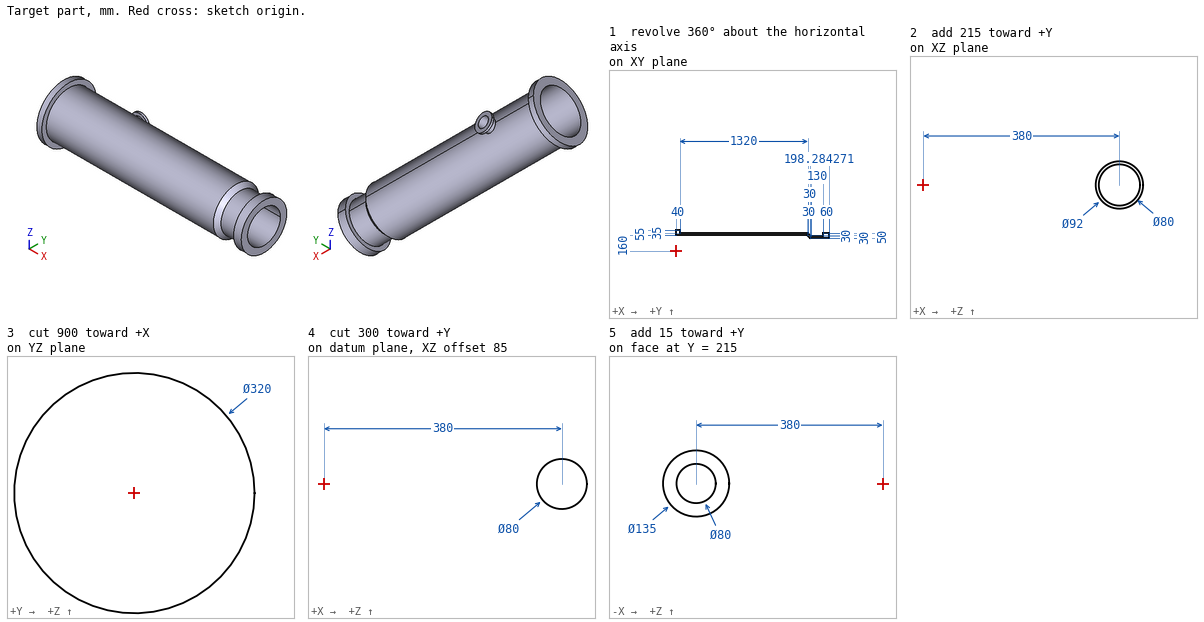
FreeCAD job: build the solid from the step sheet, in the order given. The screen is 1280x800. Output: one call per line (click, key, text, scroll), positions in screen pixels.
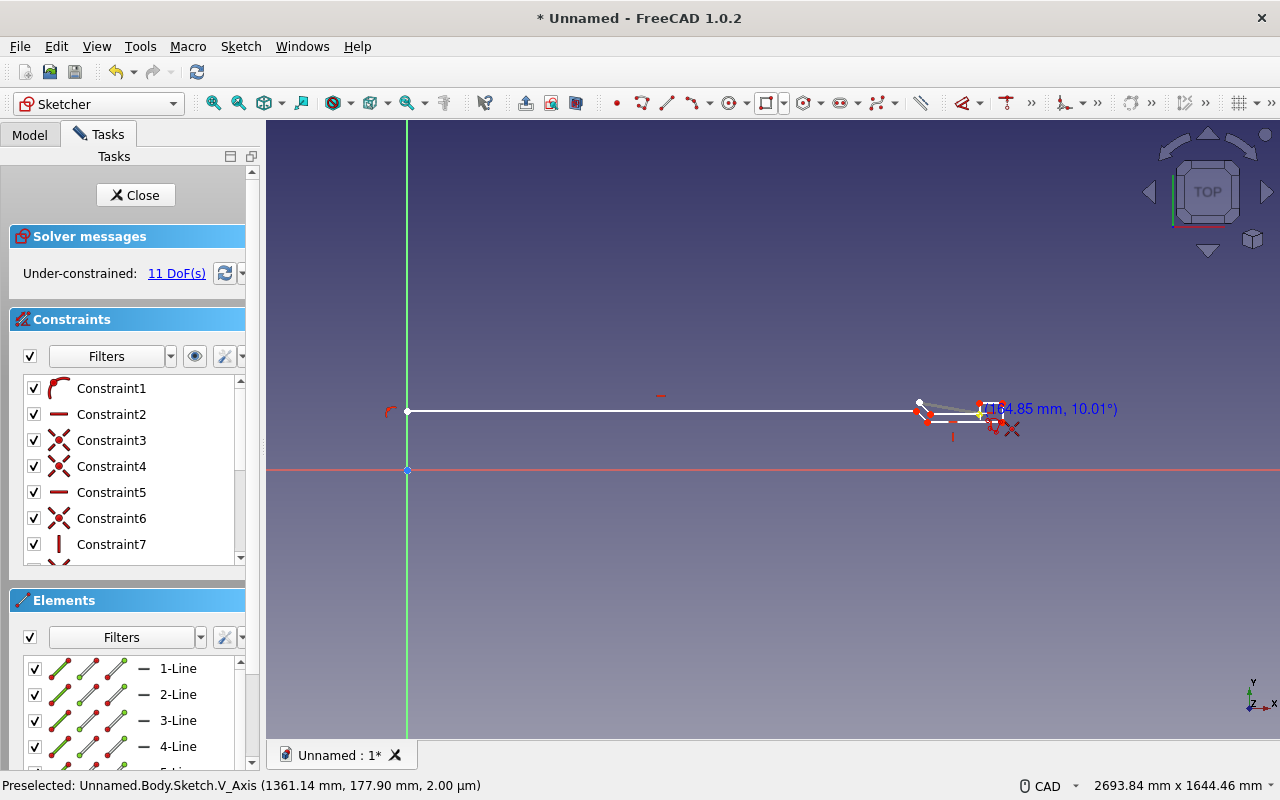
scroll(422, 403, up, 4)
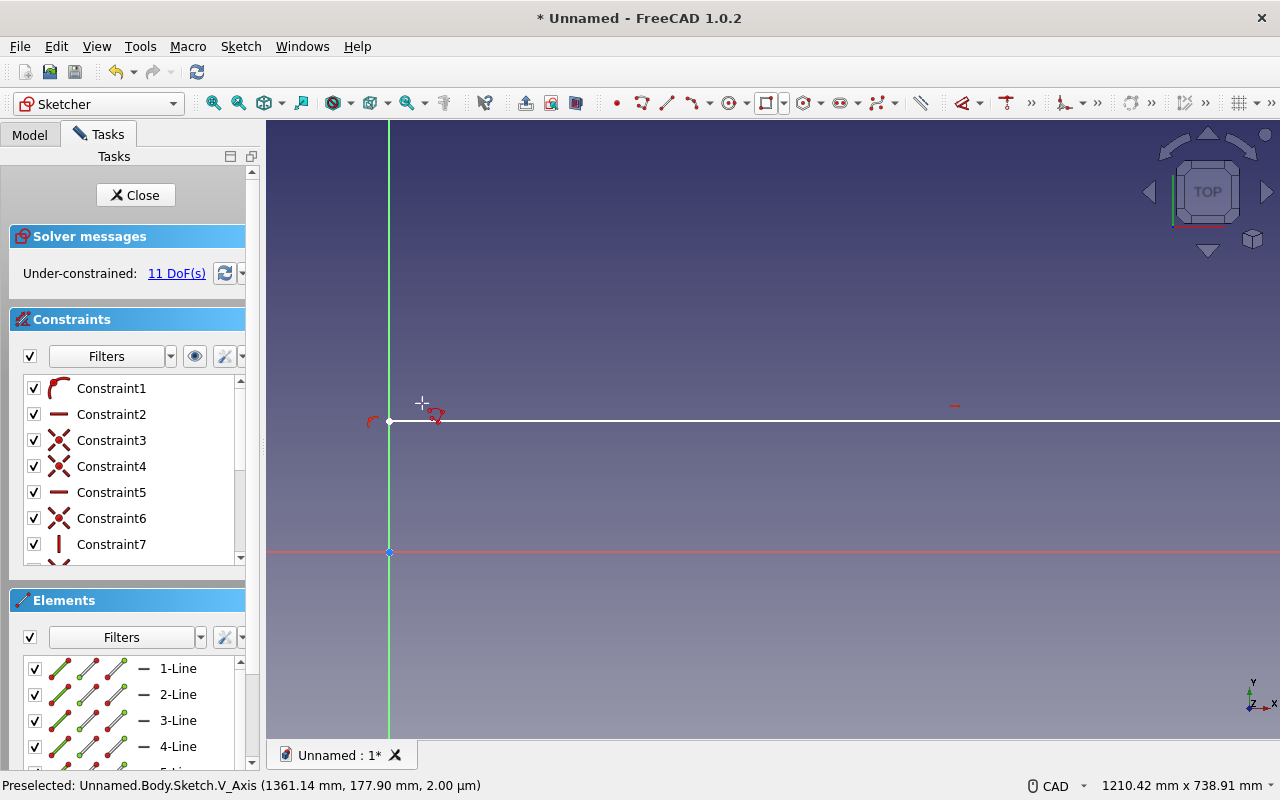
click(423, 401)
click(423, 372)
click(398, 372)
click(389, 421)
key(Escape)
key(Escape)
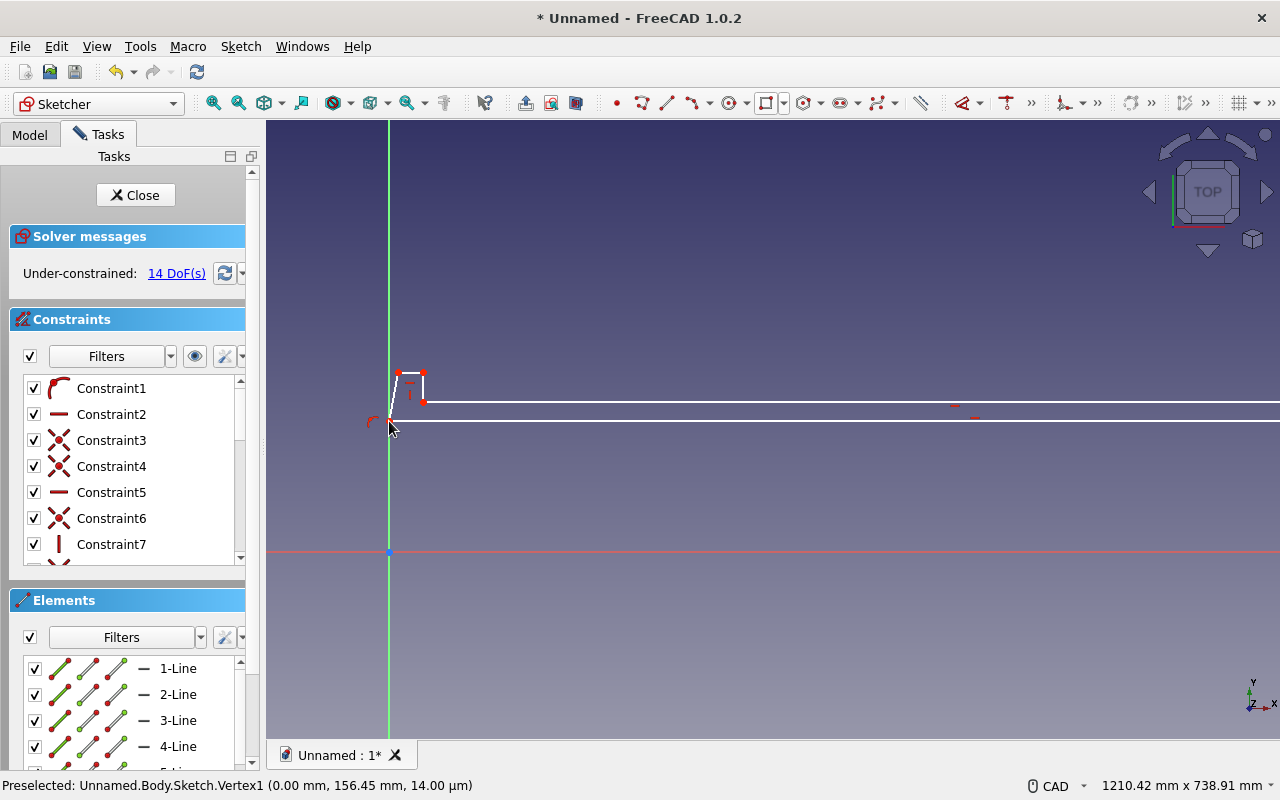
click(392, 407)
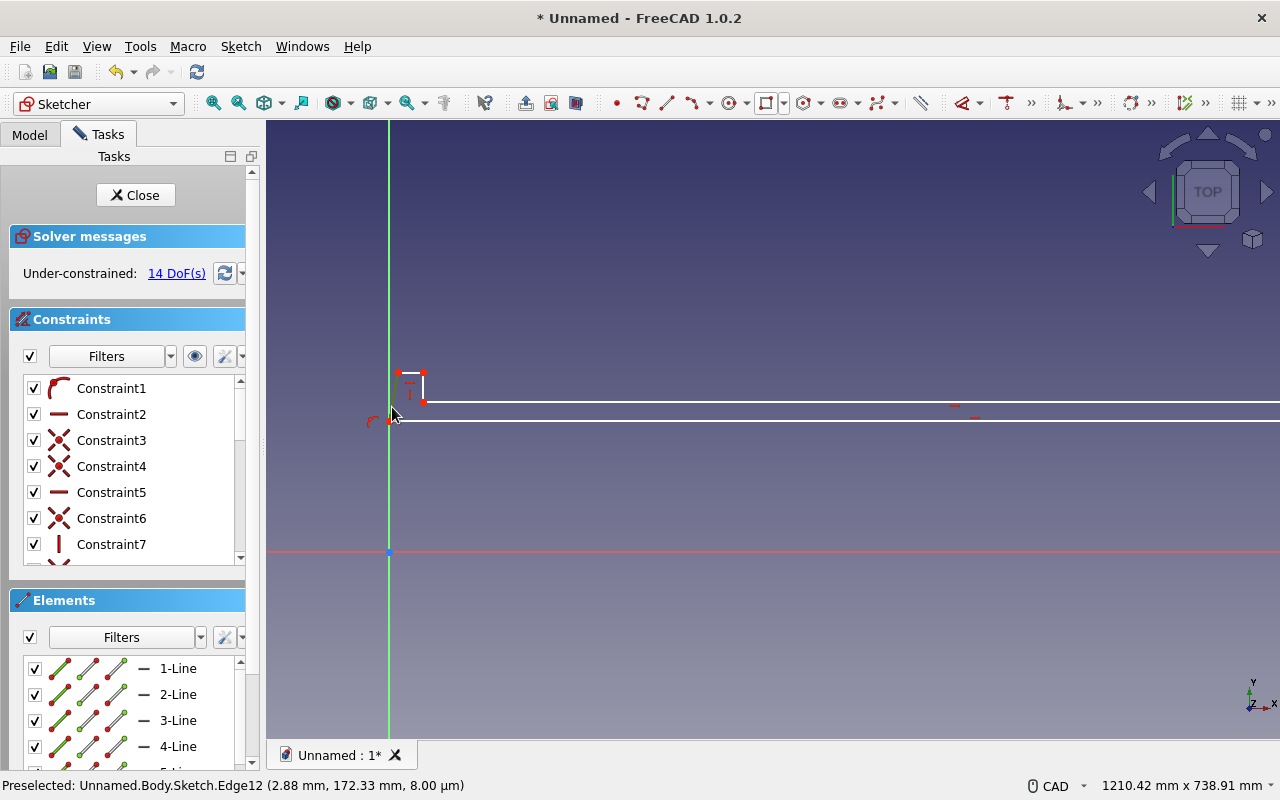
key(v)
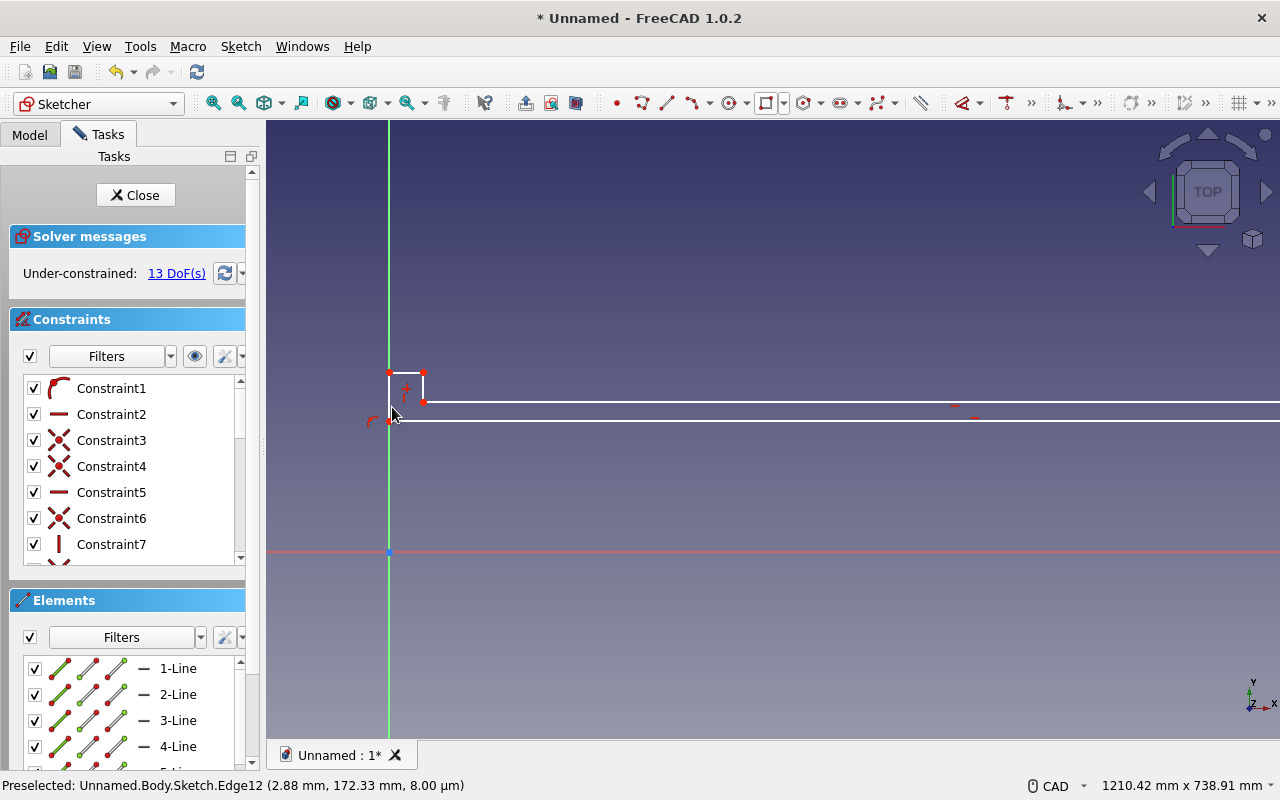
scroll(422, 403, down, 4)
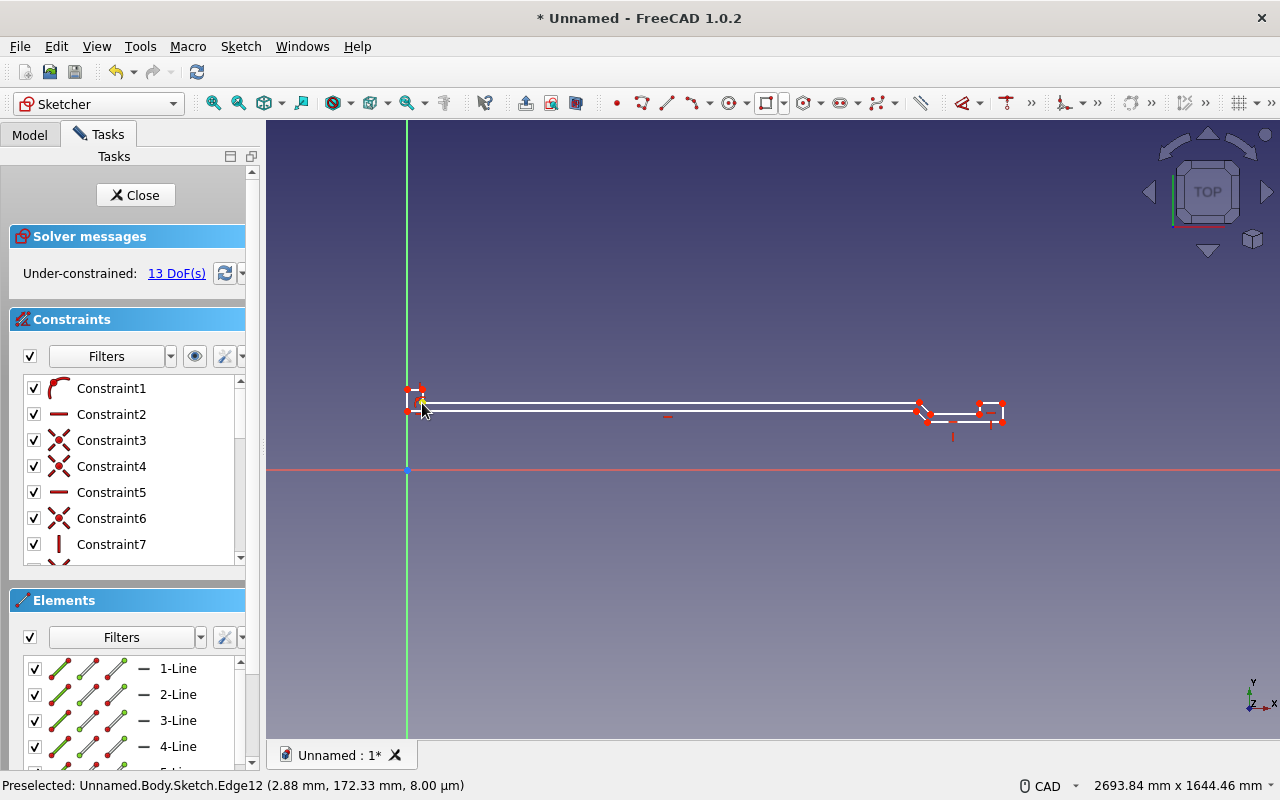
scroll(1003, 417, up, 5)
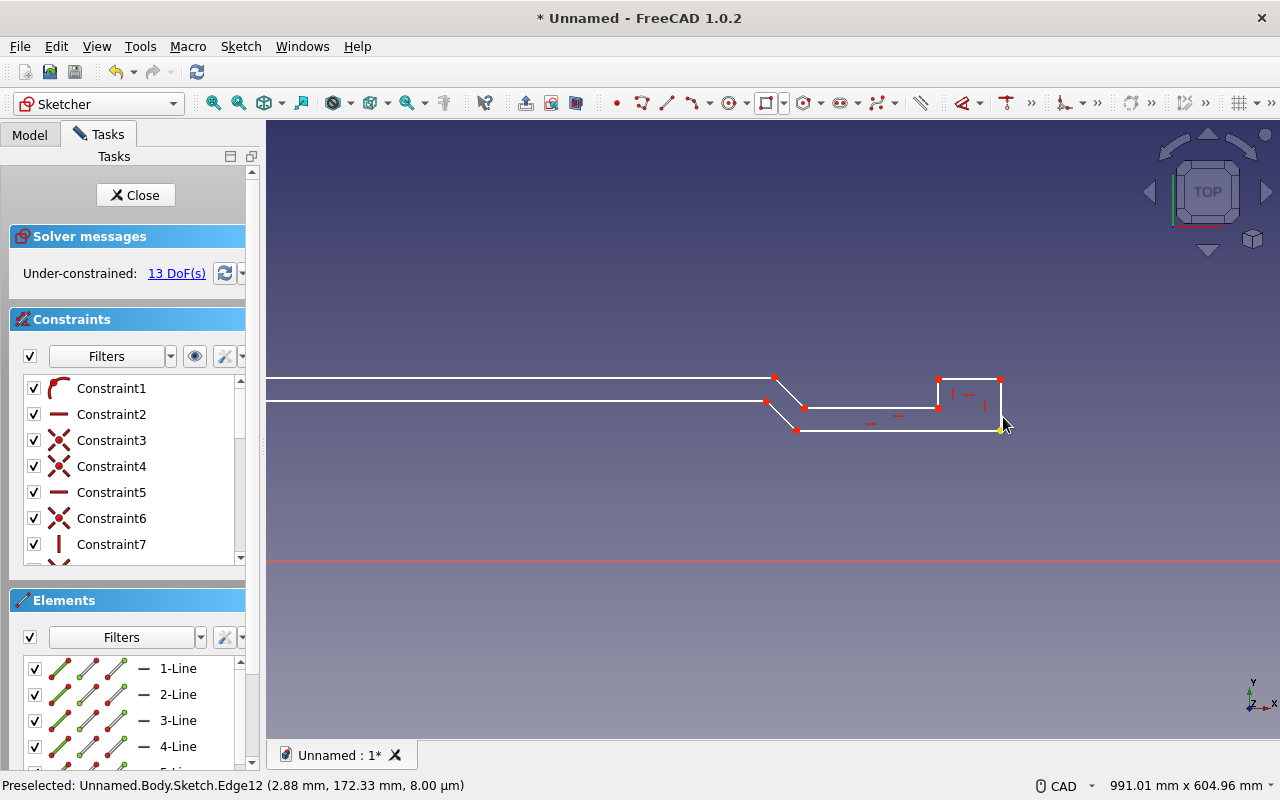
click(1001, 415)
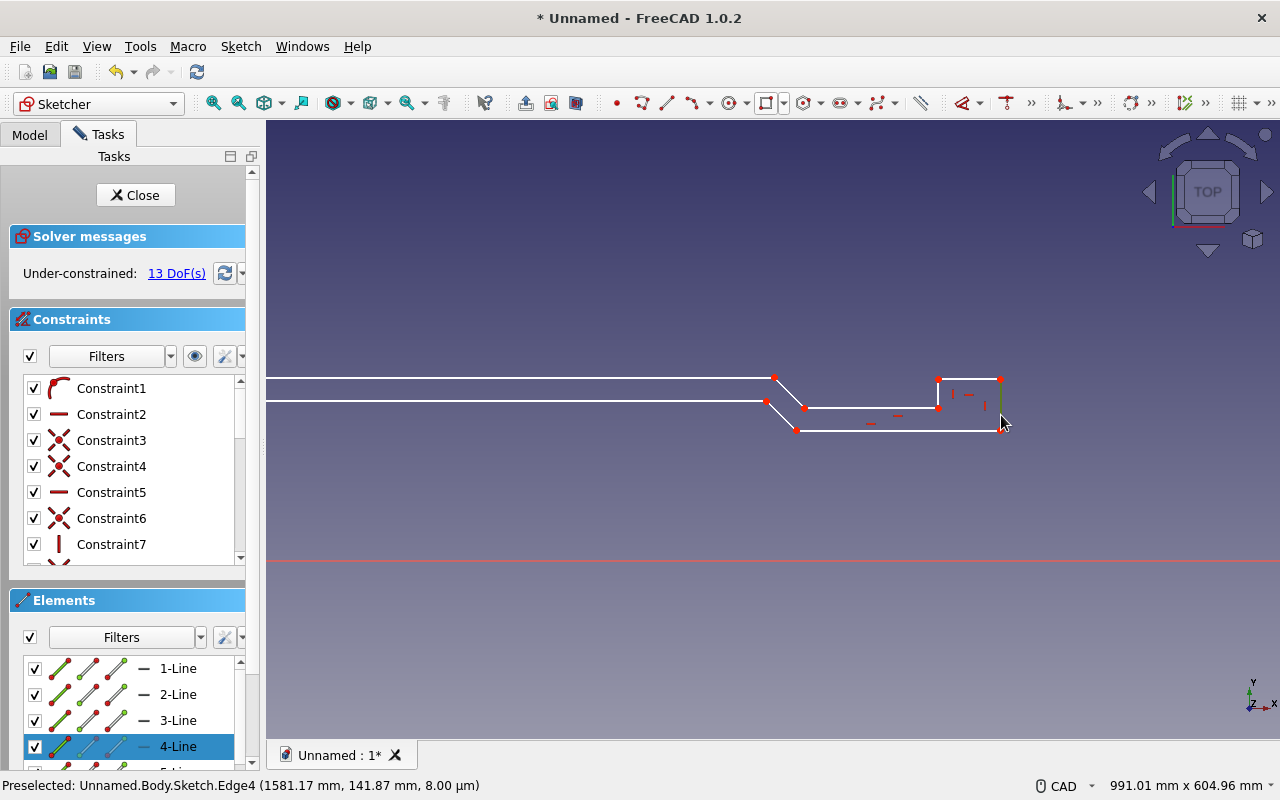
key(i)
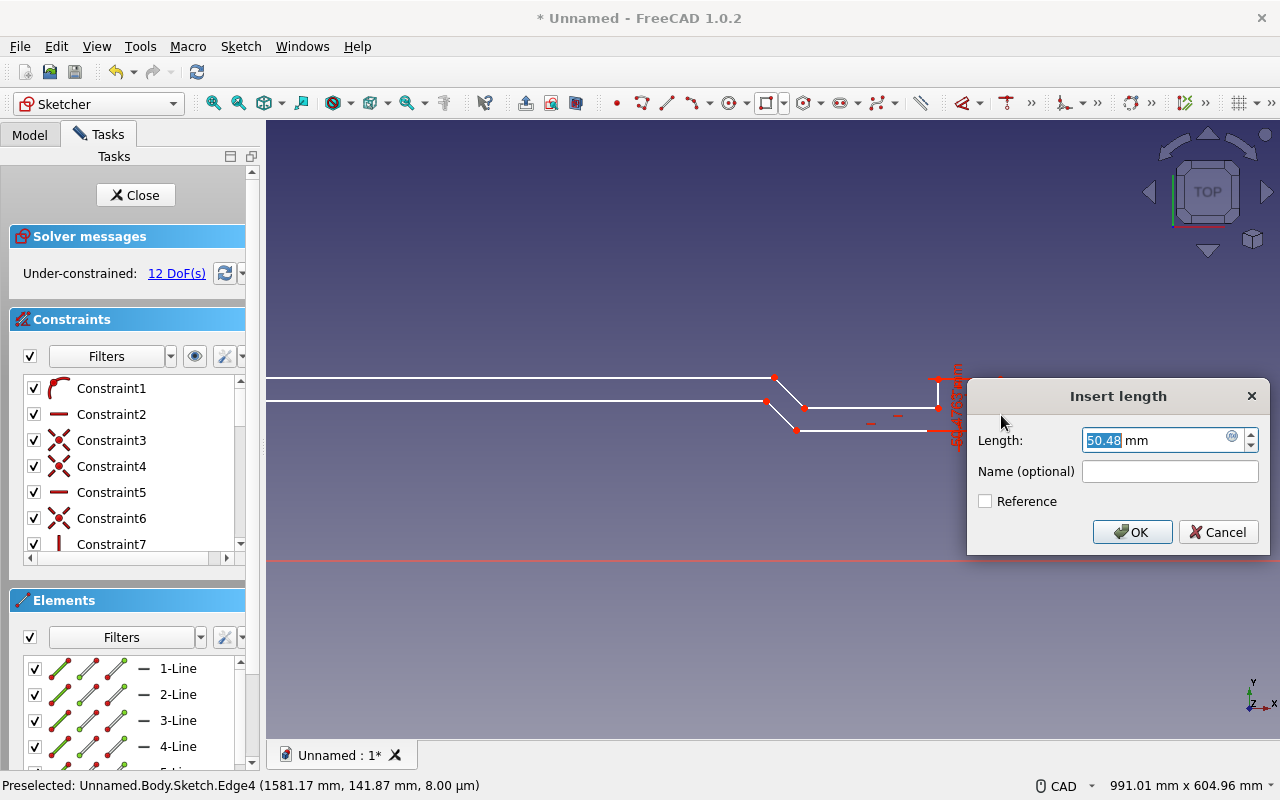
text(50)
key(Return)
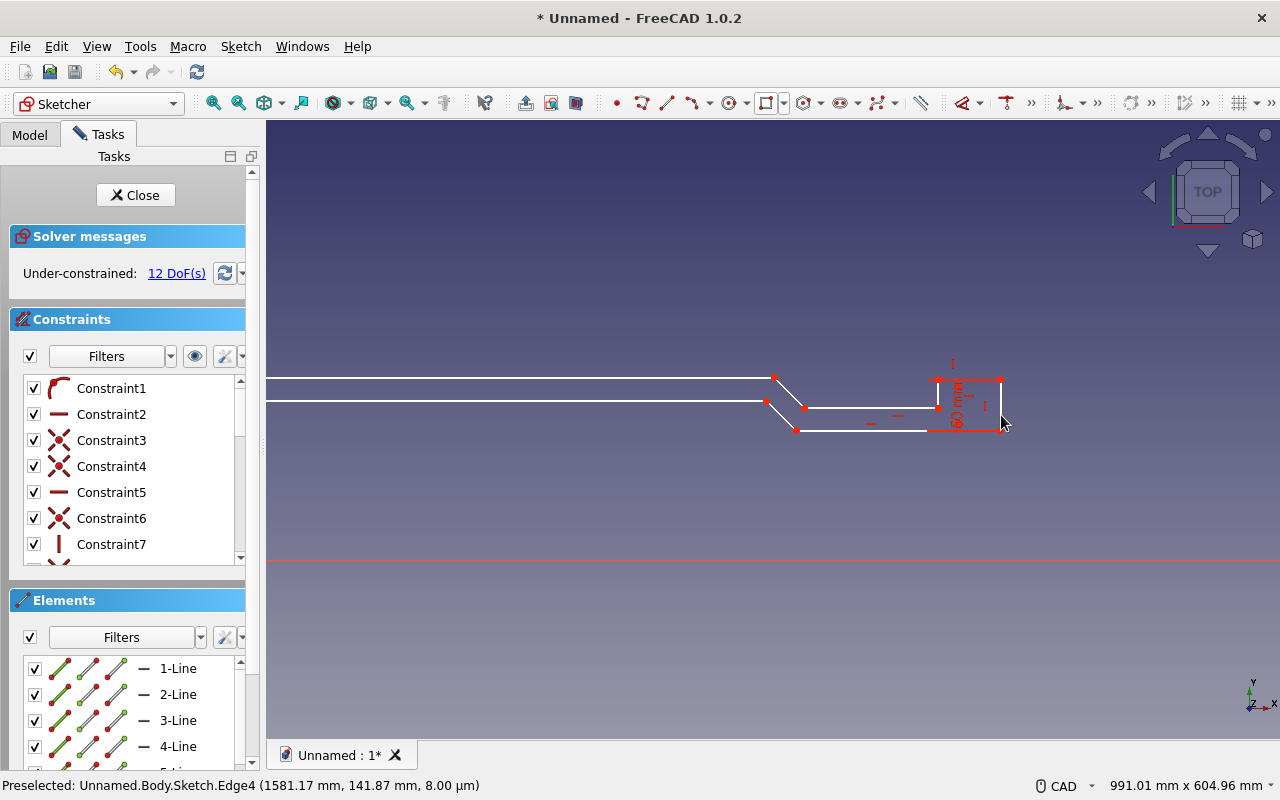
click(982, 380)